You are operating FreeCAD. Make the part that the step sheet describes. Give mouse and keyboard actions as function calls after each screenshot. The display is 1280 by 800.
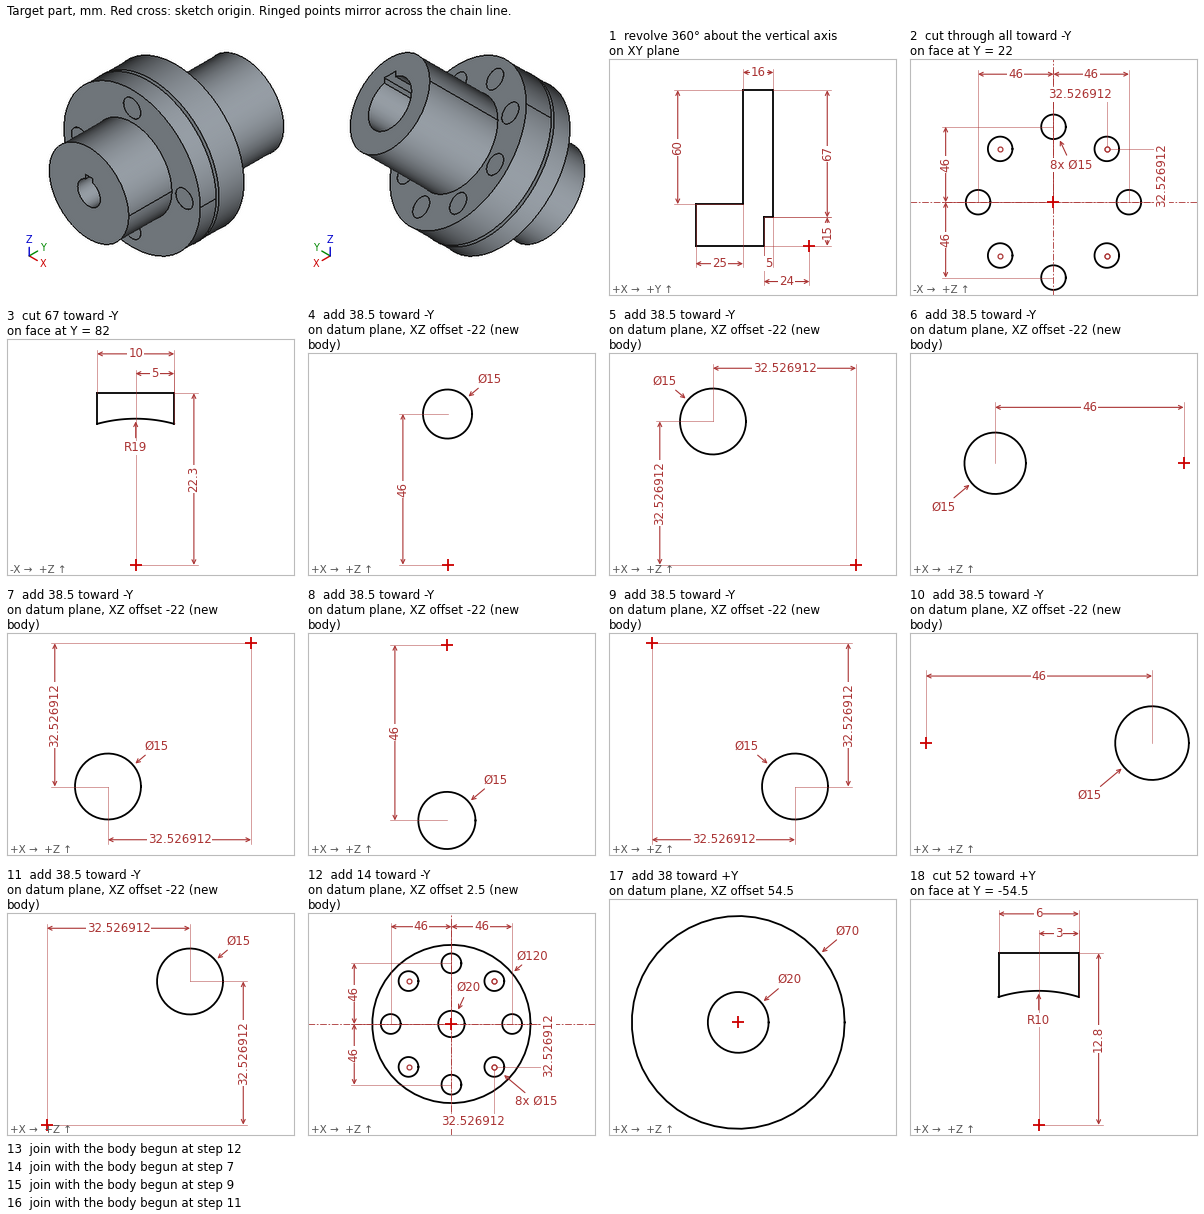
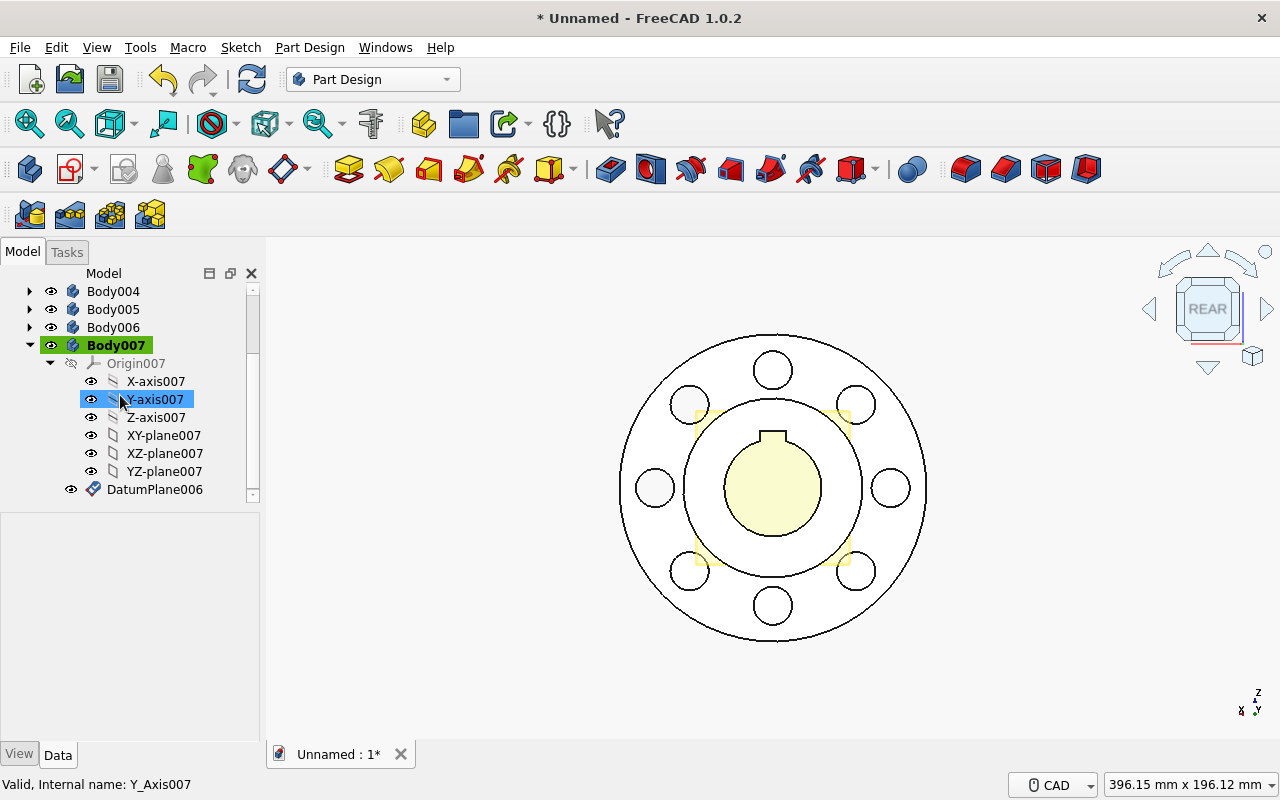
click(116, 489)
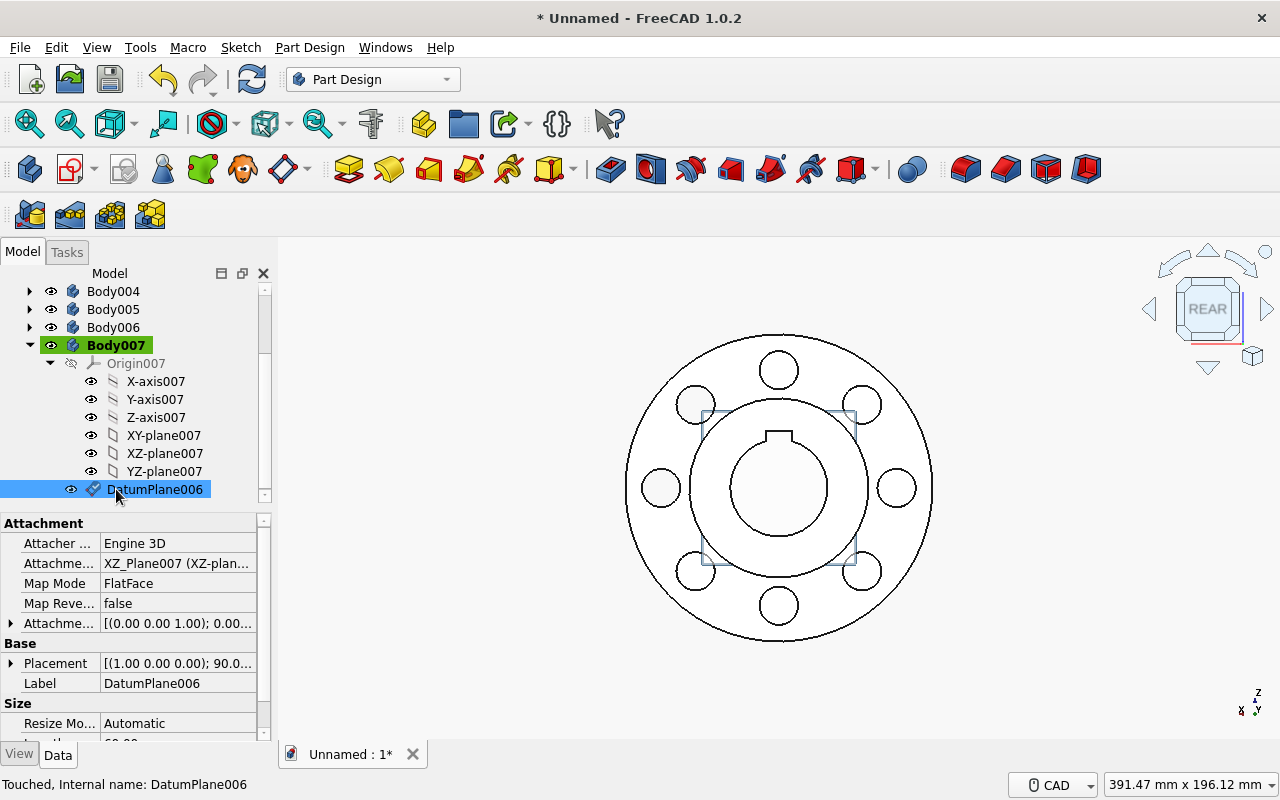
click(70, 170)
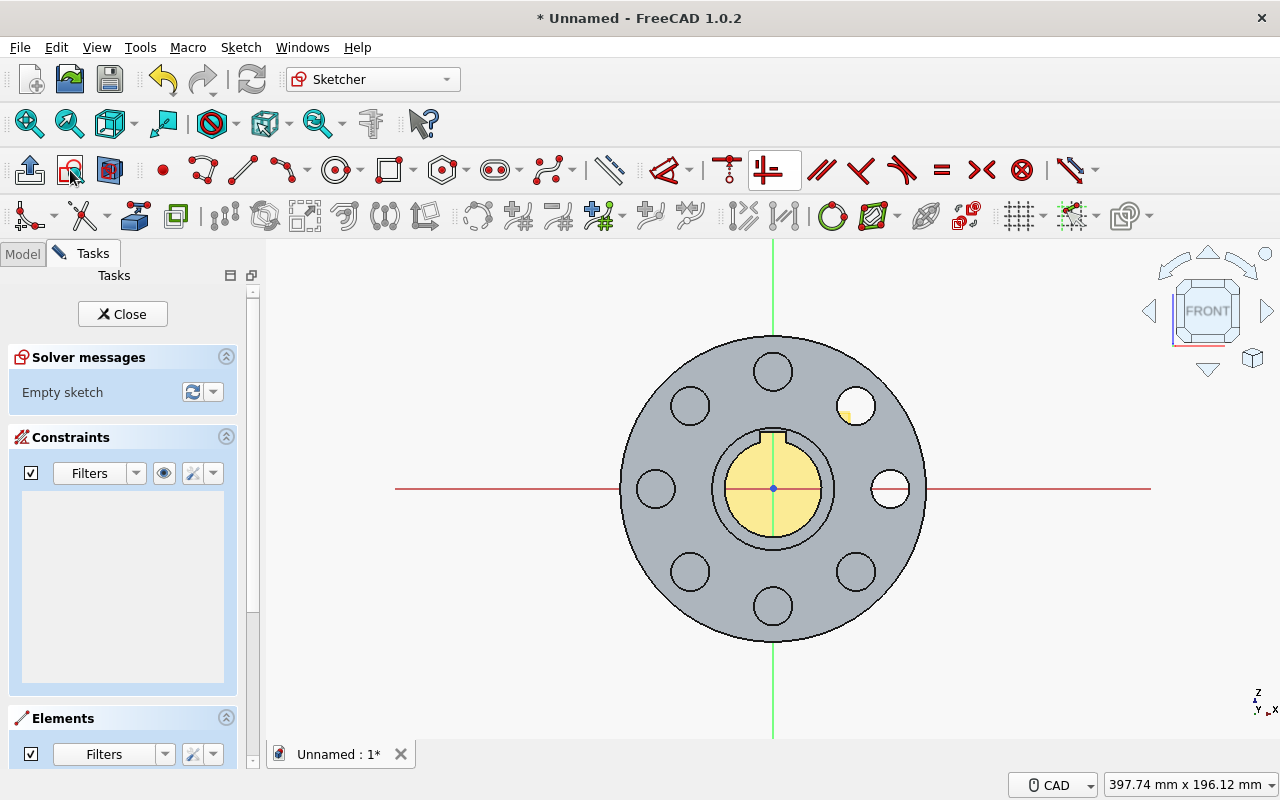
scroll(914, 489, up, 11)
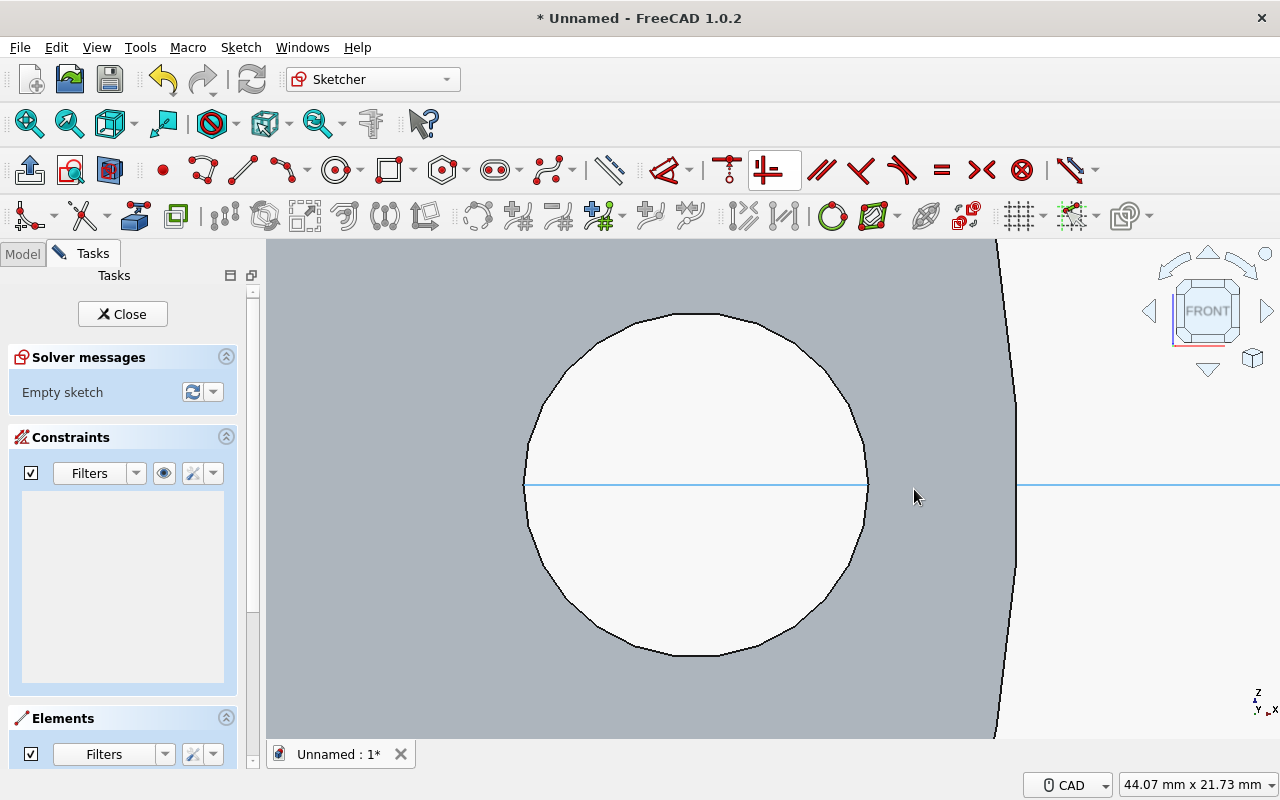
click(336, 170)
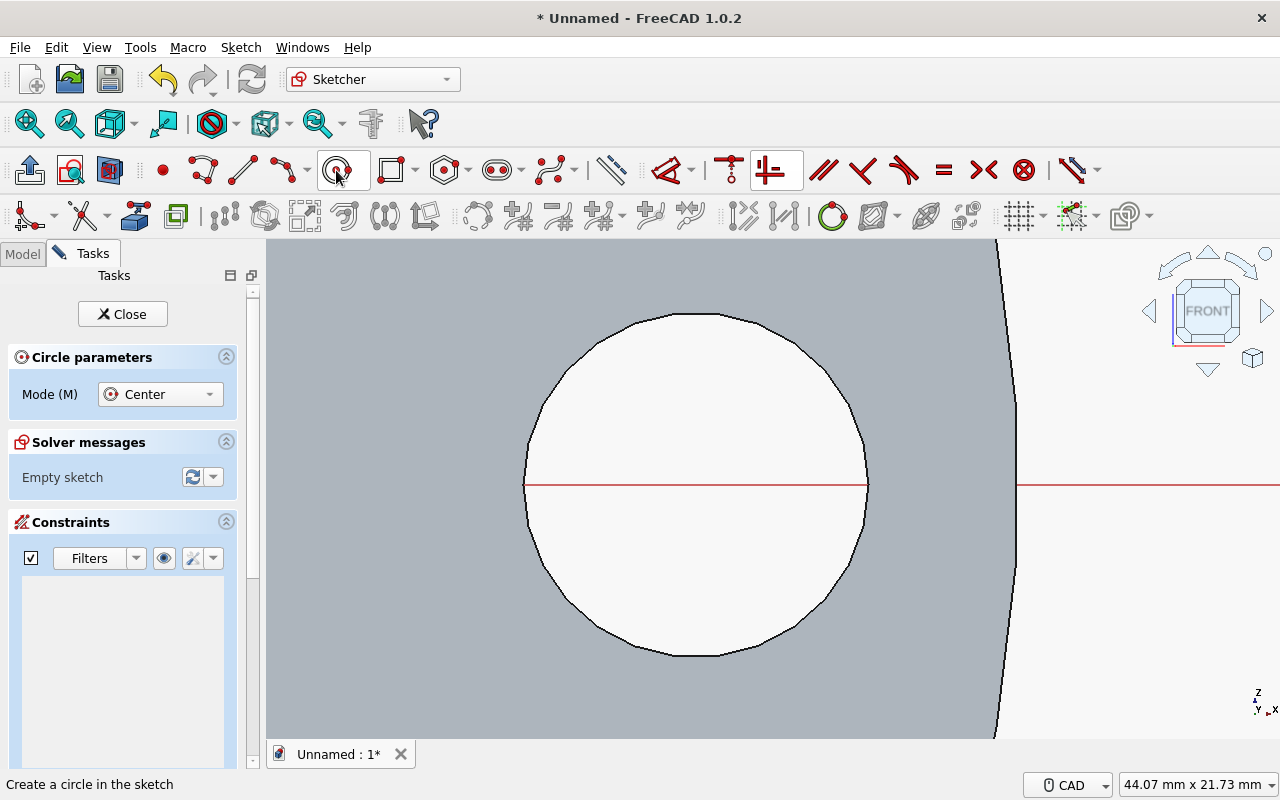
click(696, 485)
click(818, 363)
key(Escape)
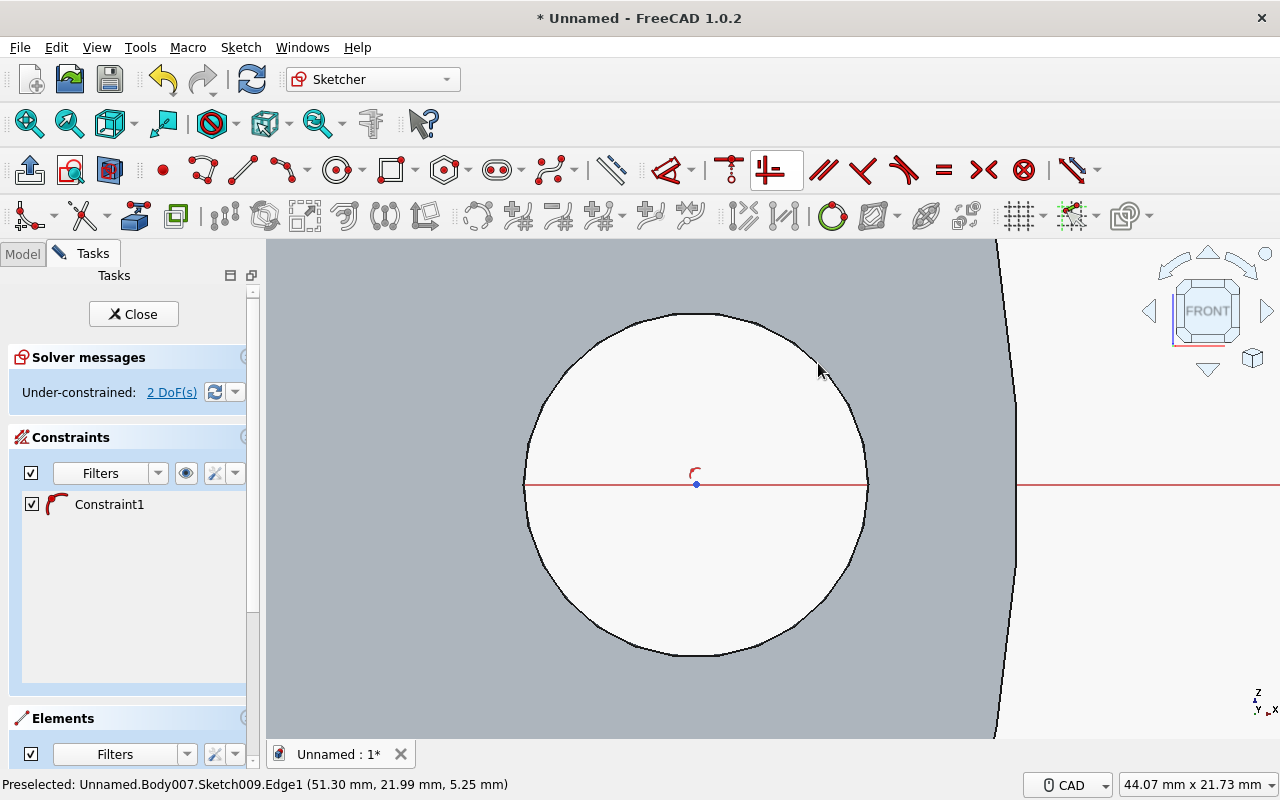
click(666, 170)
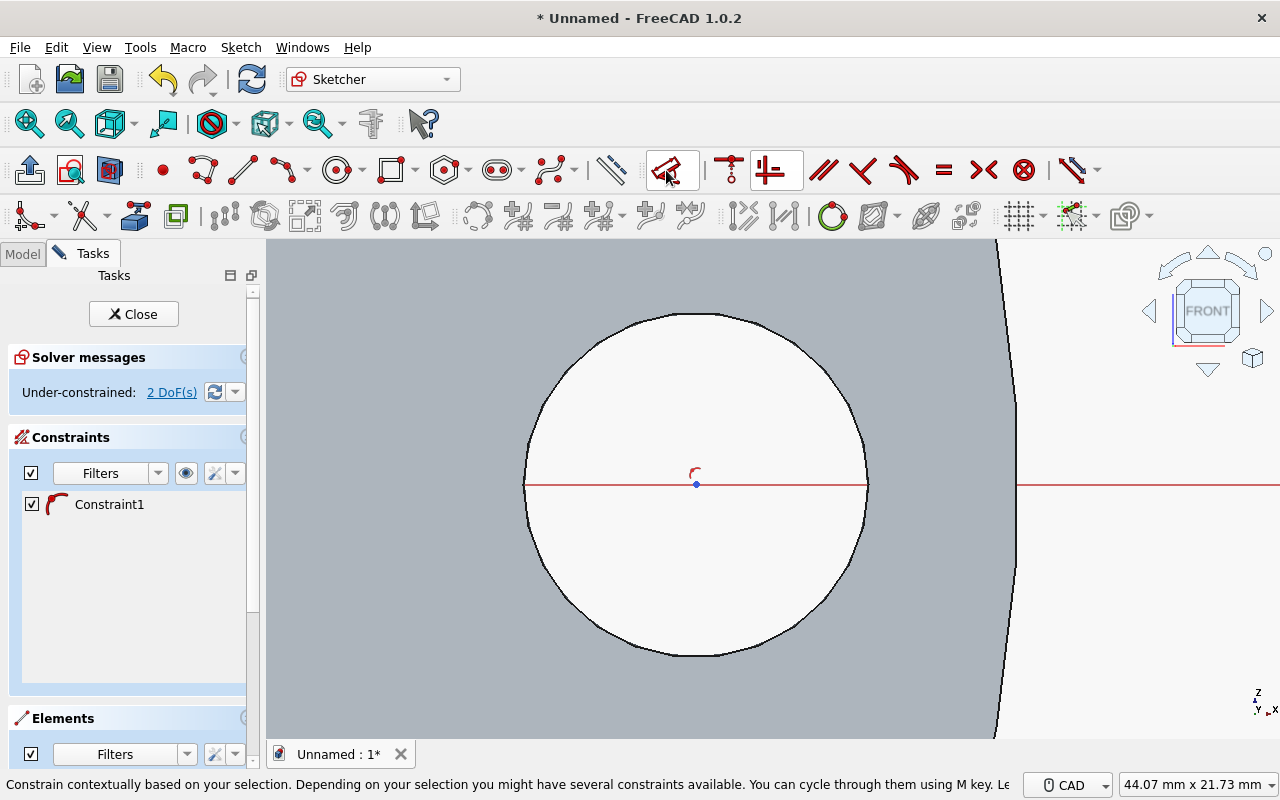
click(817, 363)
click(840, 340)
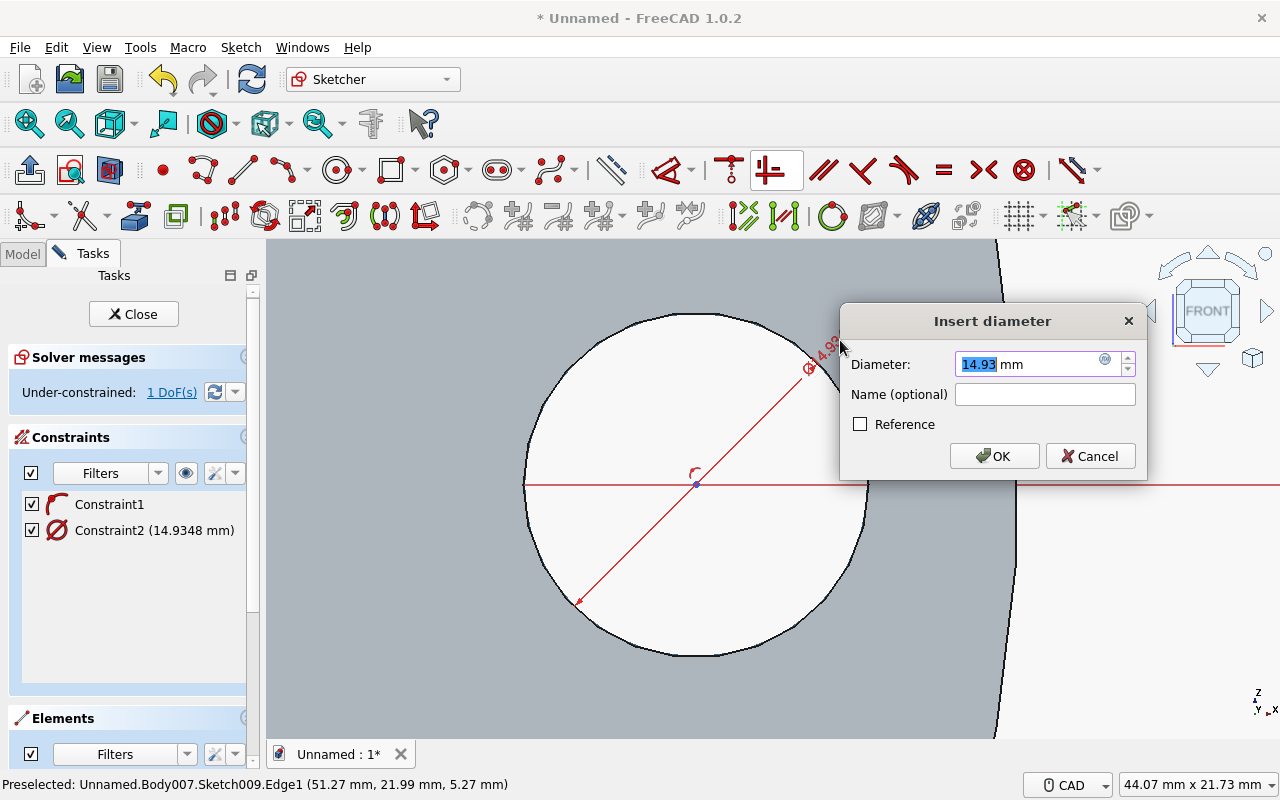
text(15)
key(Return)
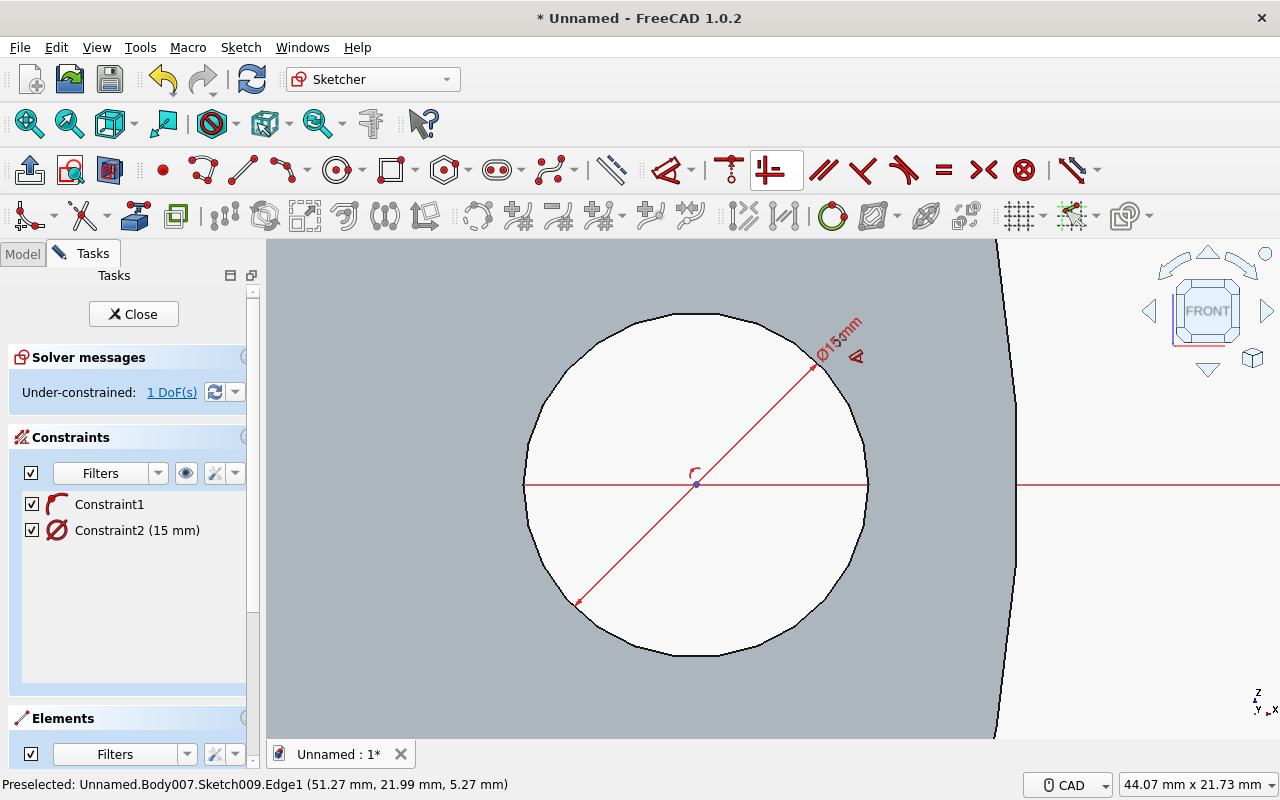
click(696, 485)
click(495, 519)